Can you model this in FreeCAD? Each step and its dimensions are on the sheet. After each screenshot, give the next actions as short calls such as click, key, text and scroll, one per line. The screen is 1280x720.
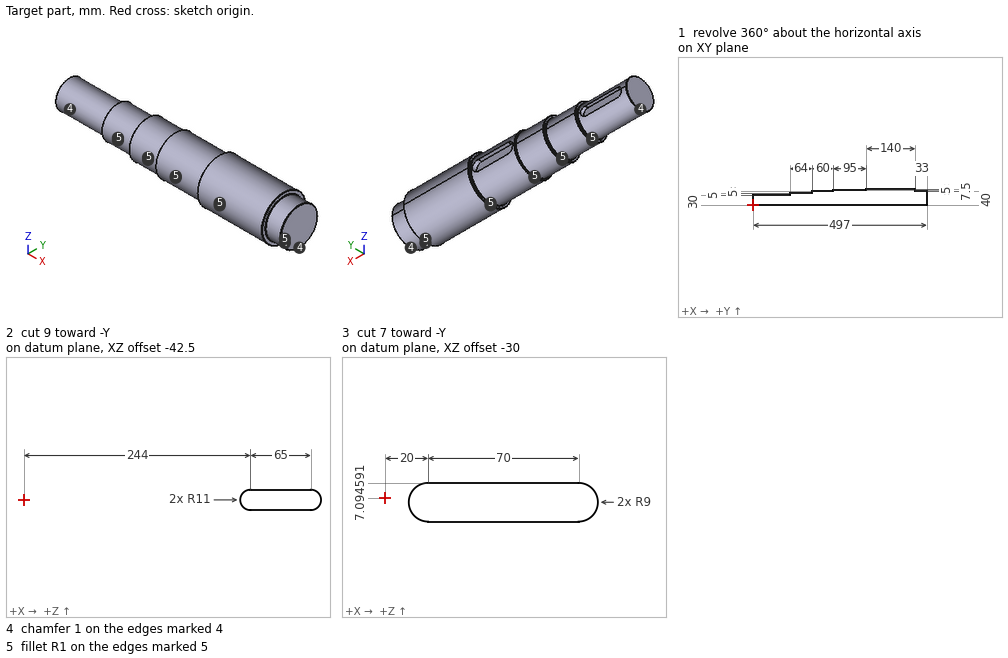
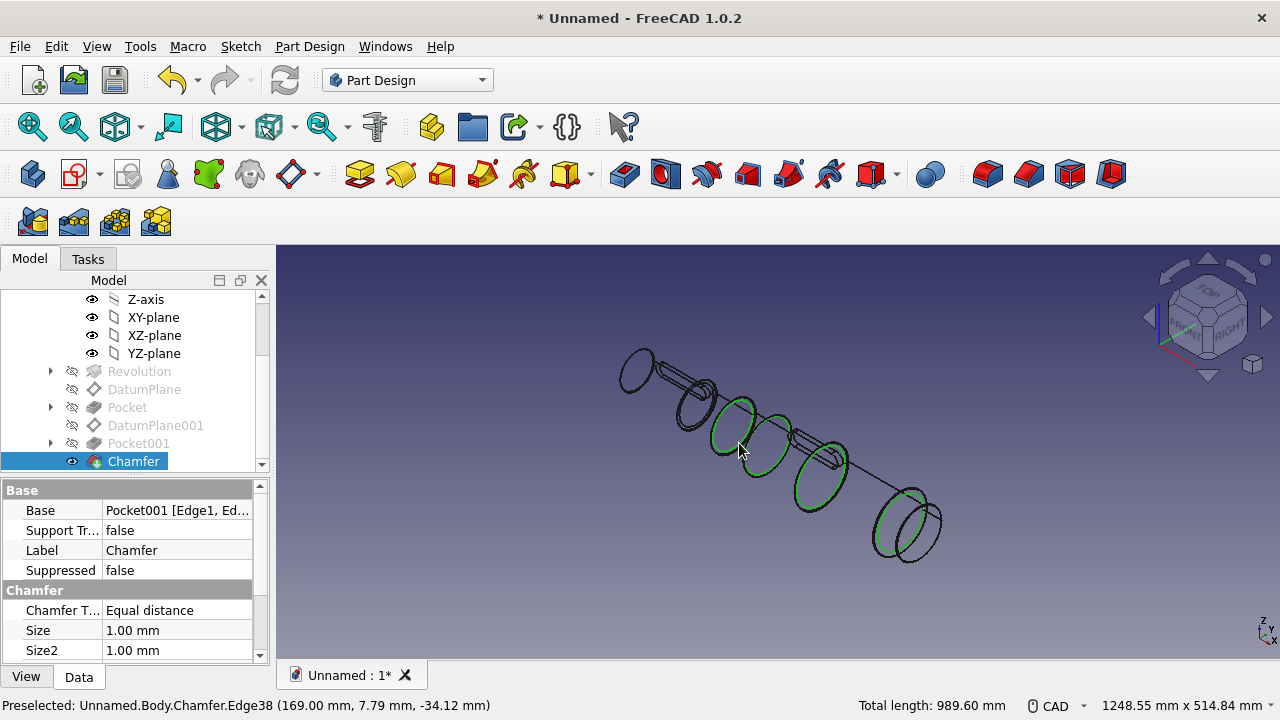
click(702, 420, ctrl)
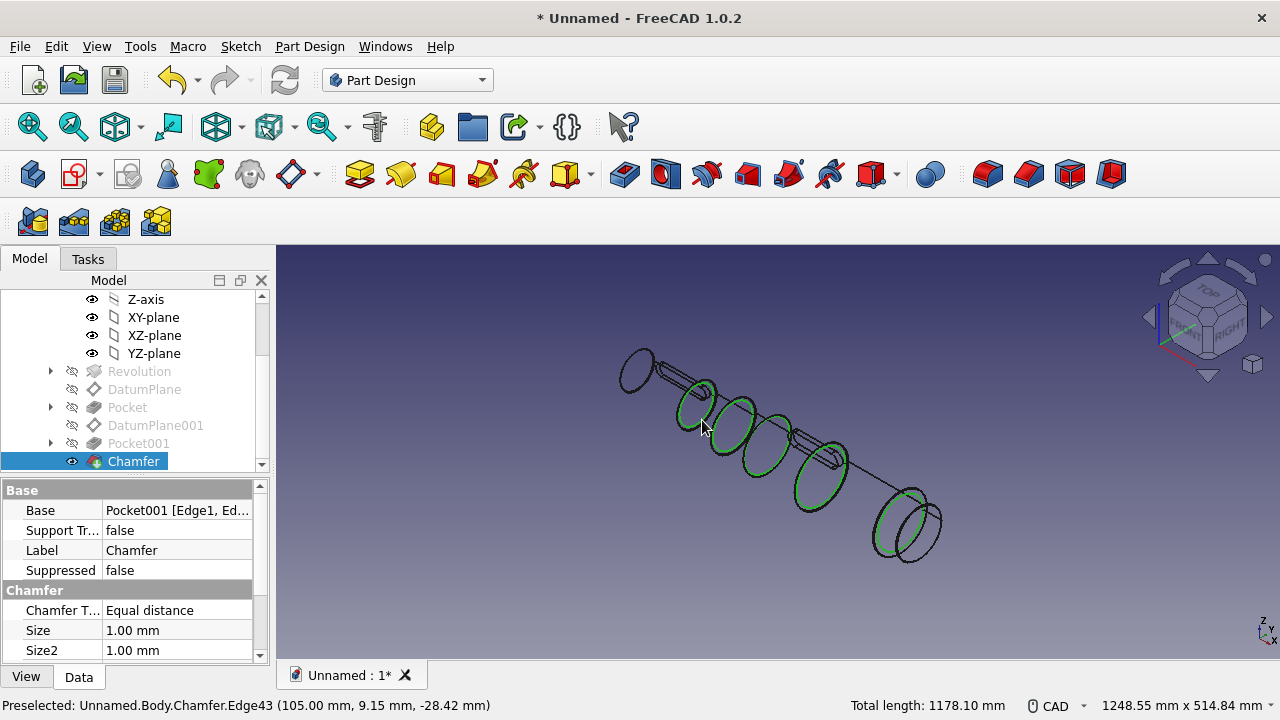
key(v)
key(1)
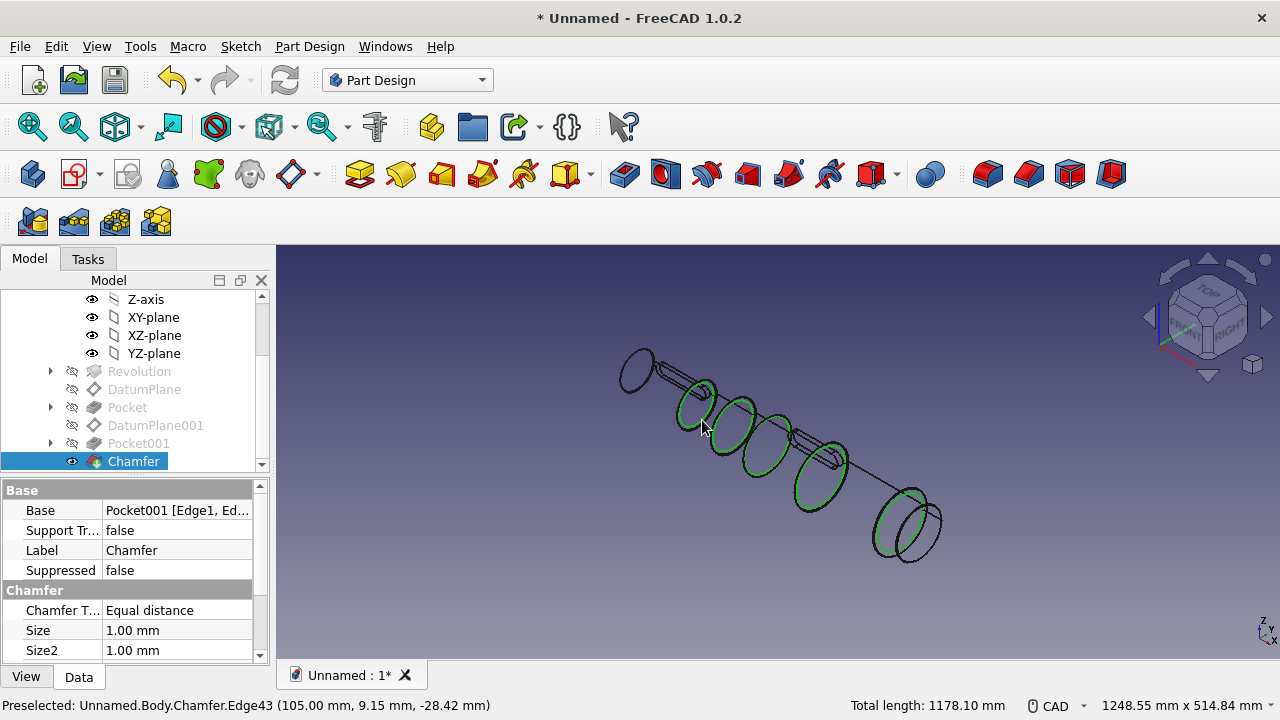
click(988, 174)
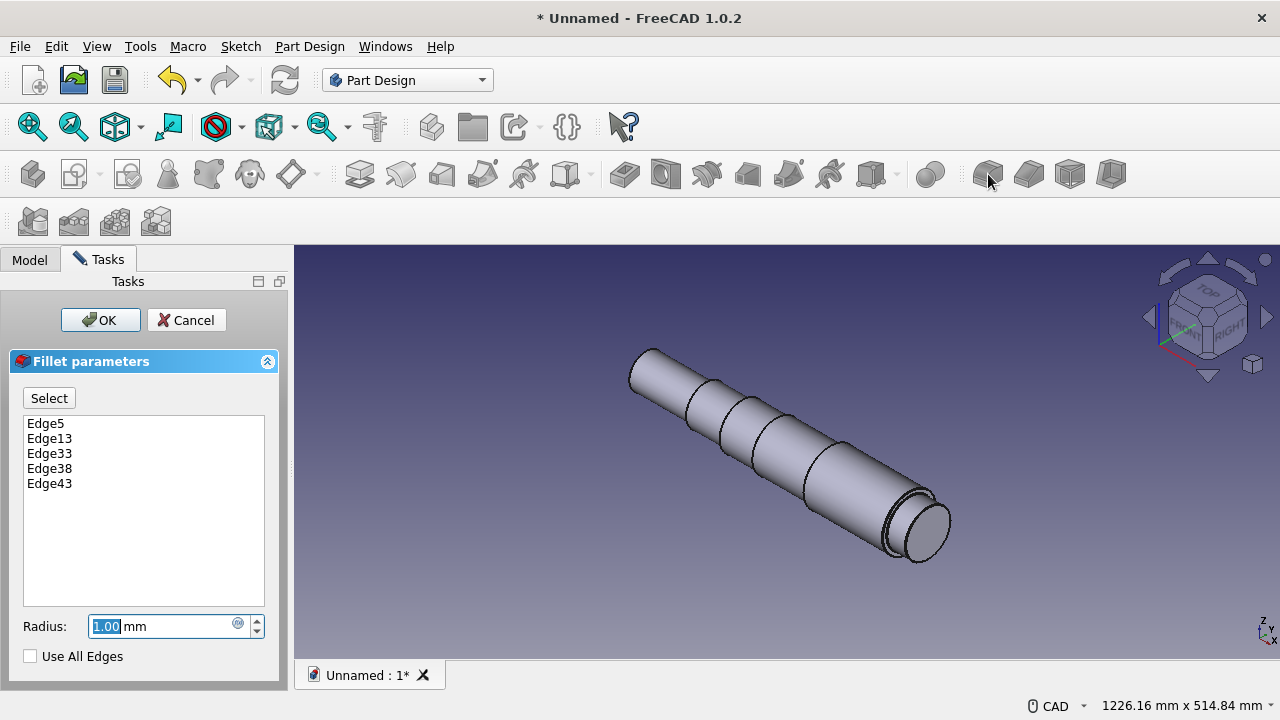
text(1)
key(Tab)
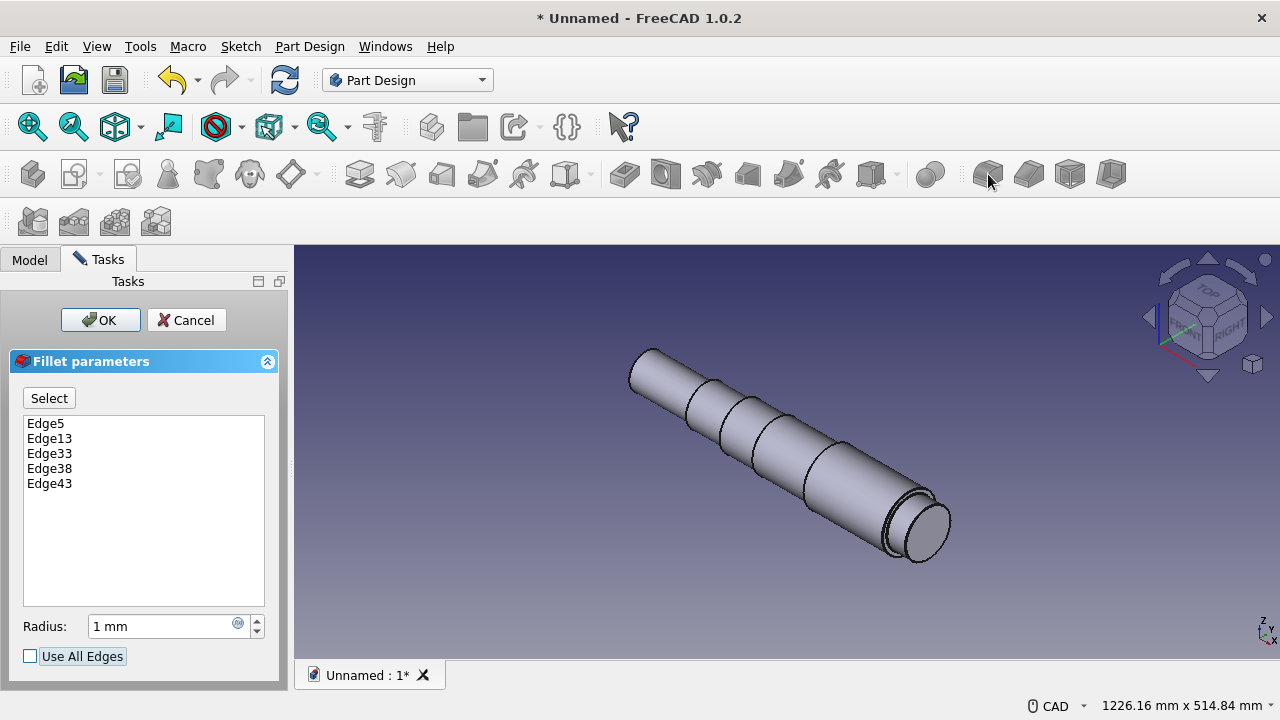
click(101, 320)